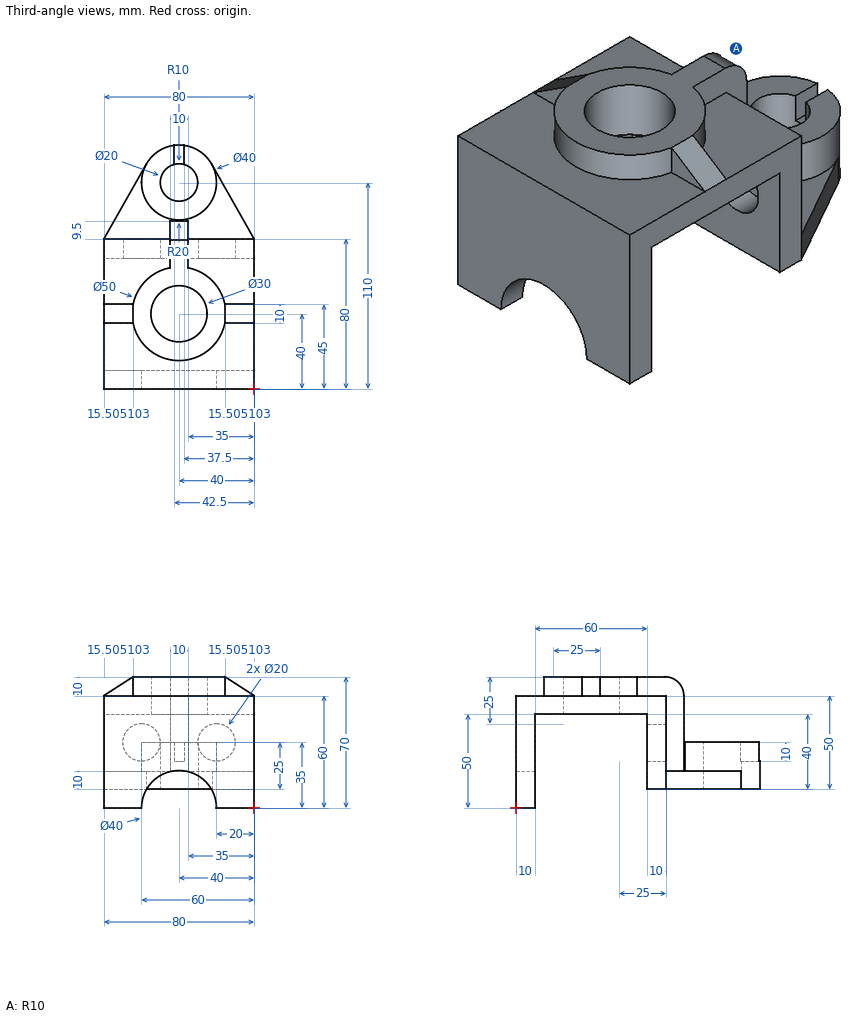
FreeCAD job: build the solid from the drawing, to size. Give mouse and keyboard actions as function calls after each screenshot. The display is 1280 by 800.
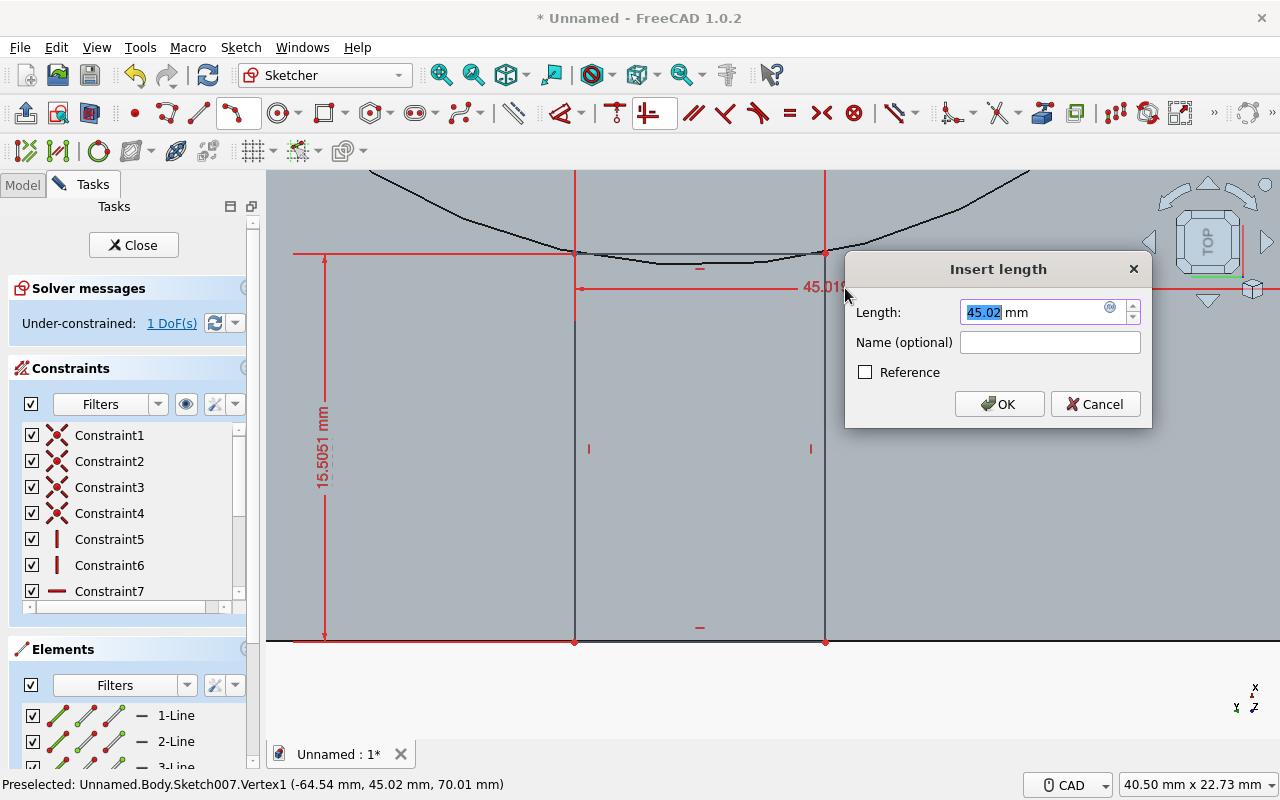
text(45)
key(Return)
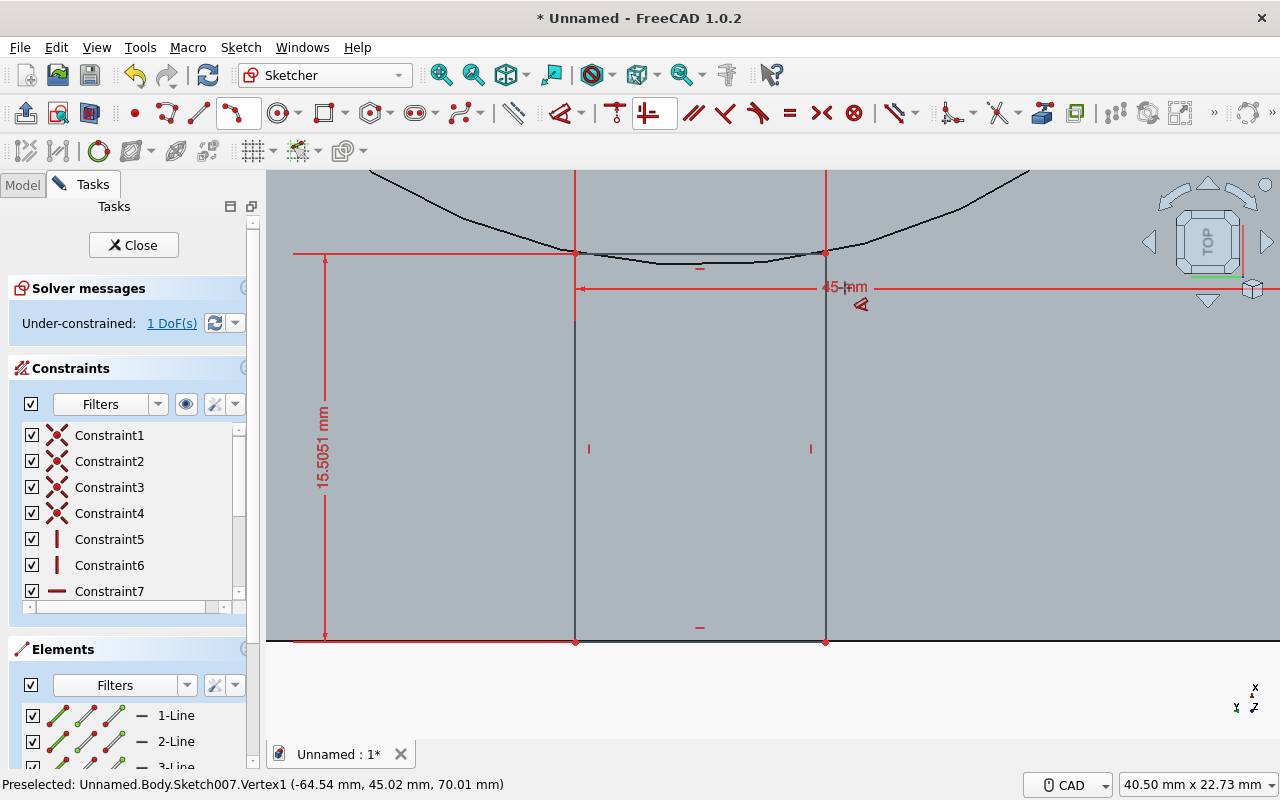
click(575, 642)
click(541, 420)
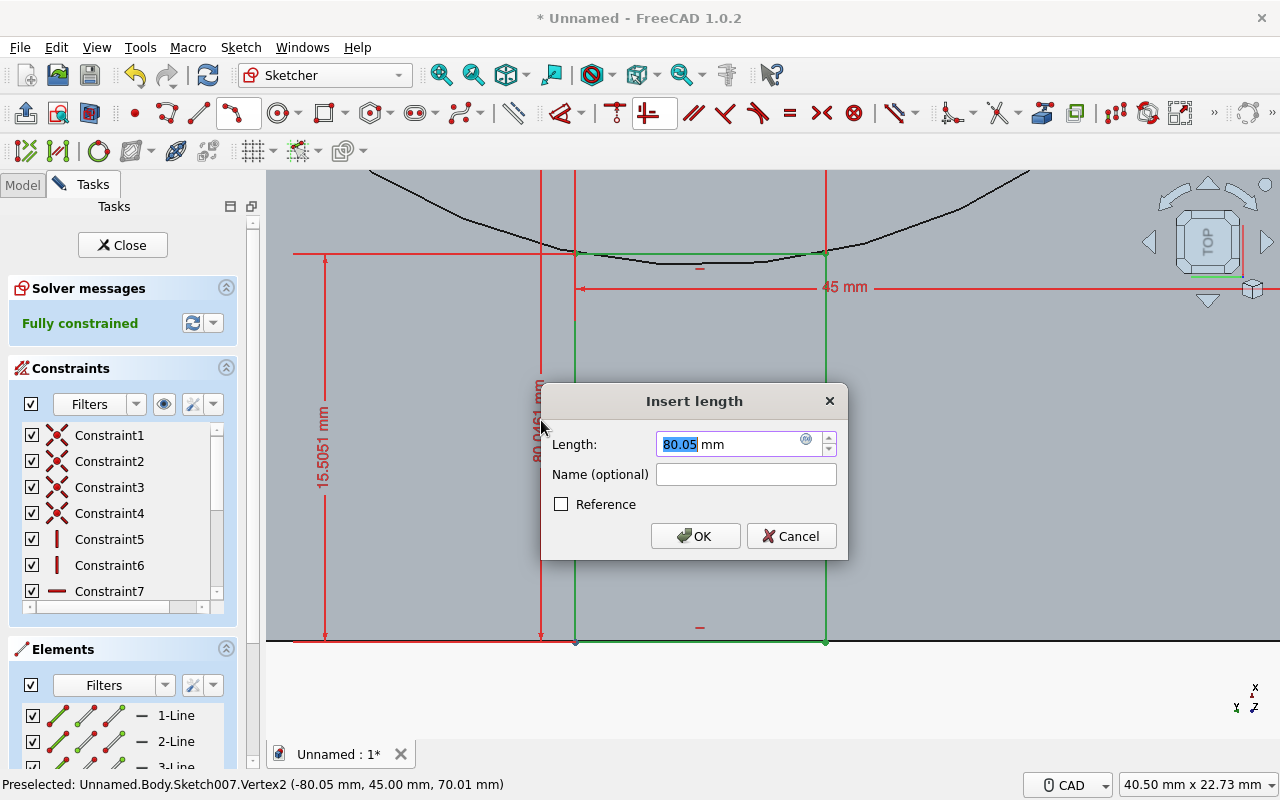
text(80)
key(Return)
key(Escape)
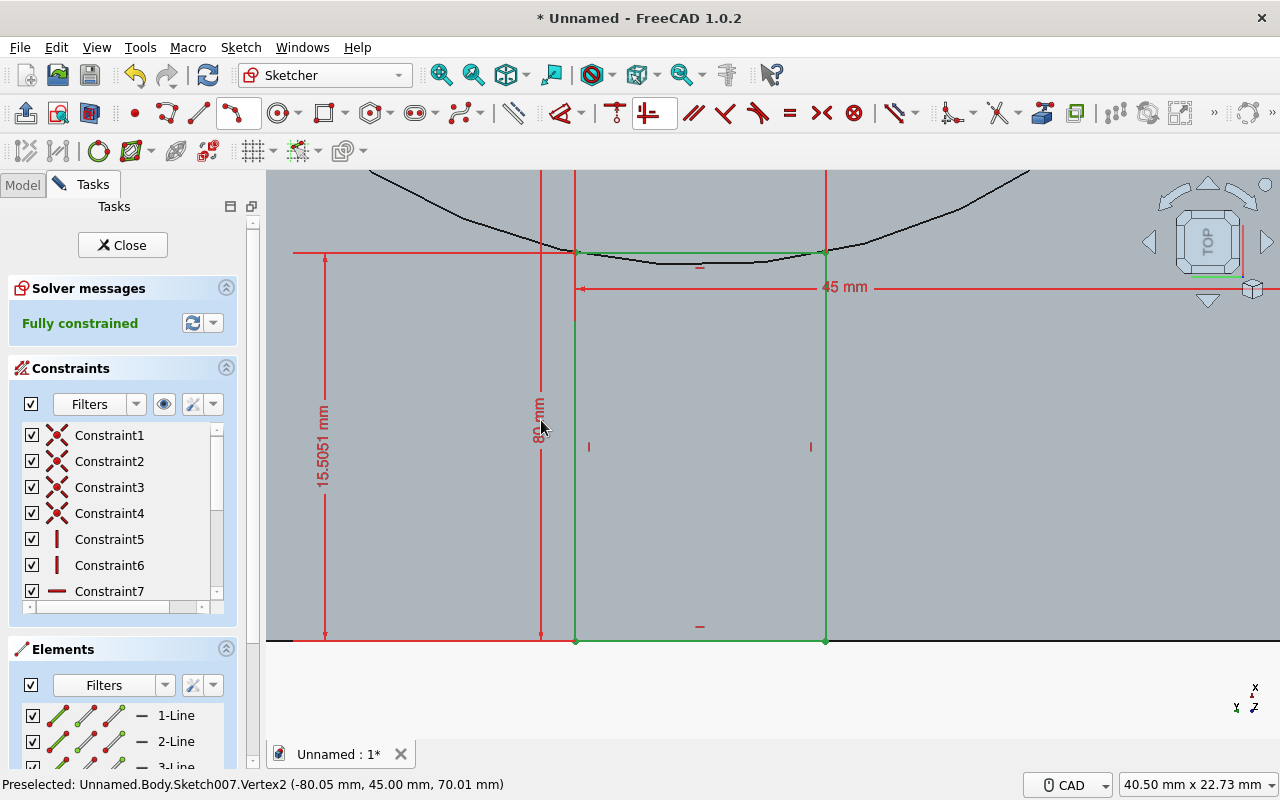
click(123, 245)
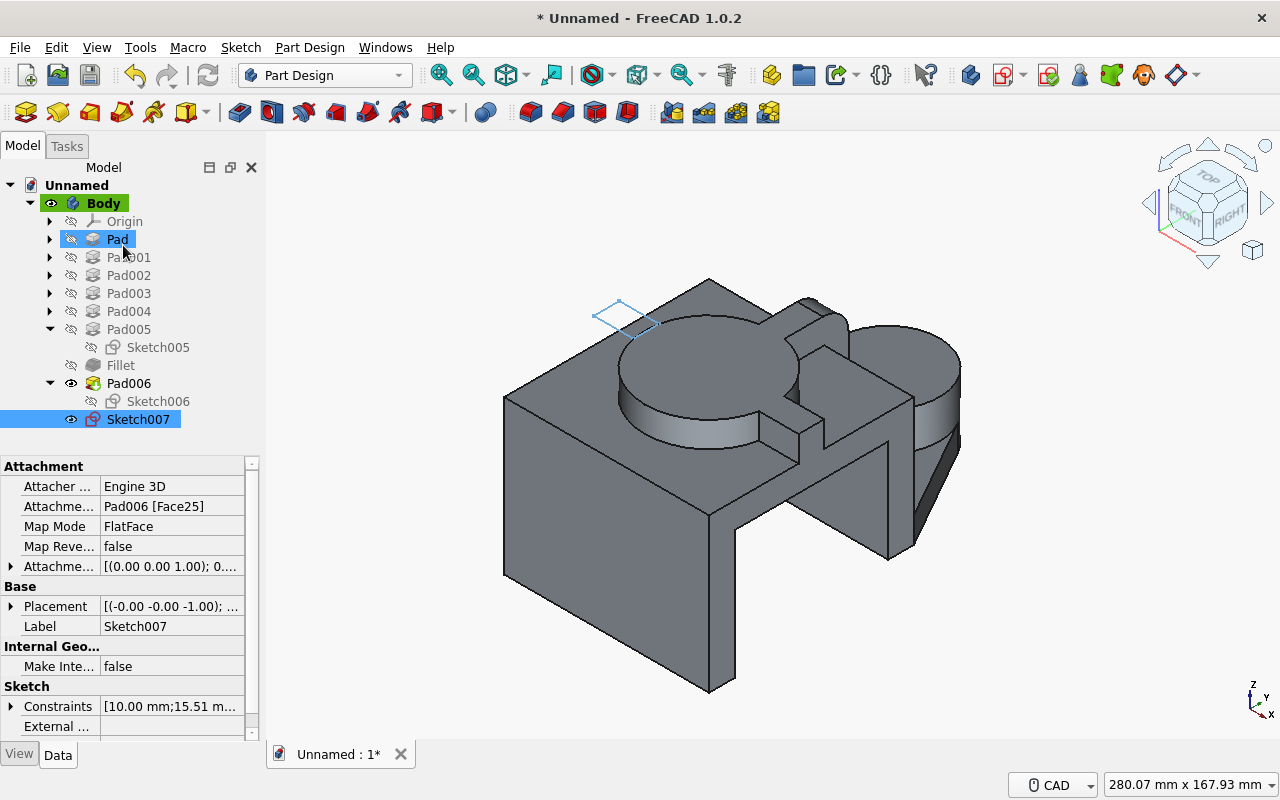
click(26, 112)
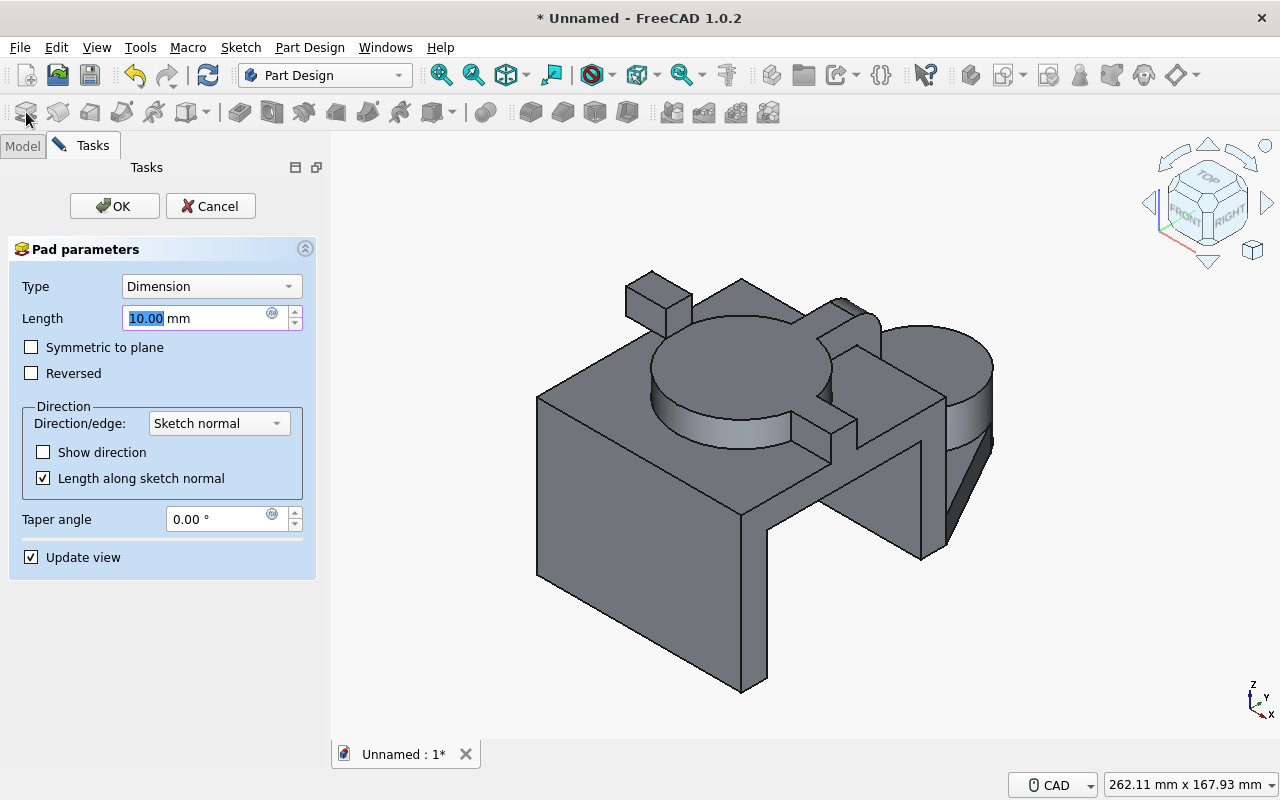
click(212, 286)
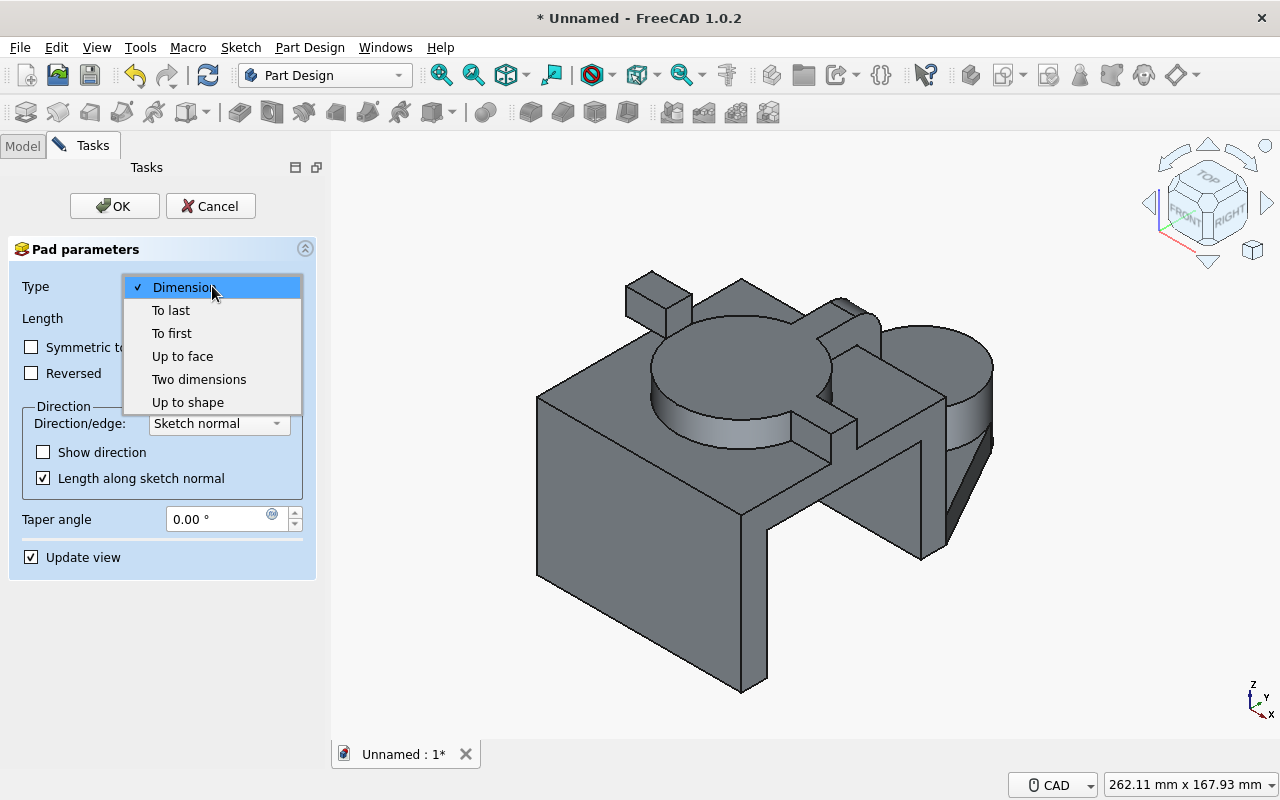
click(212, 334)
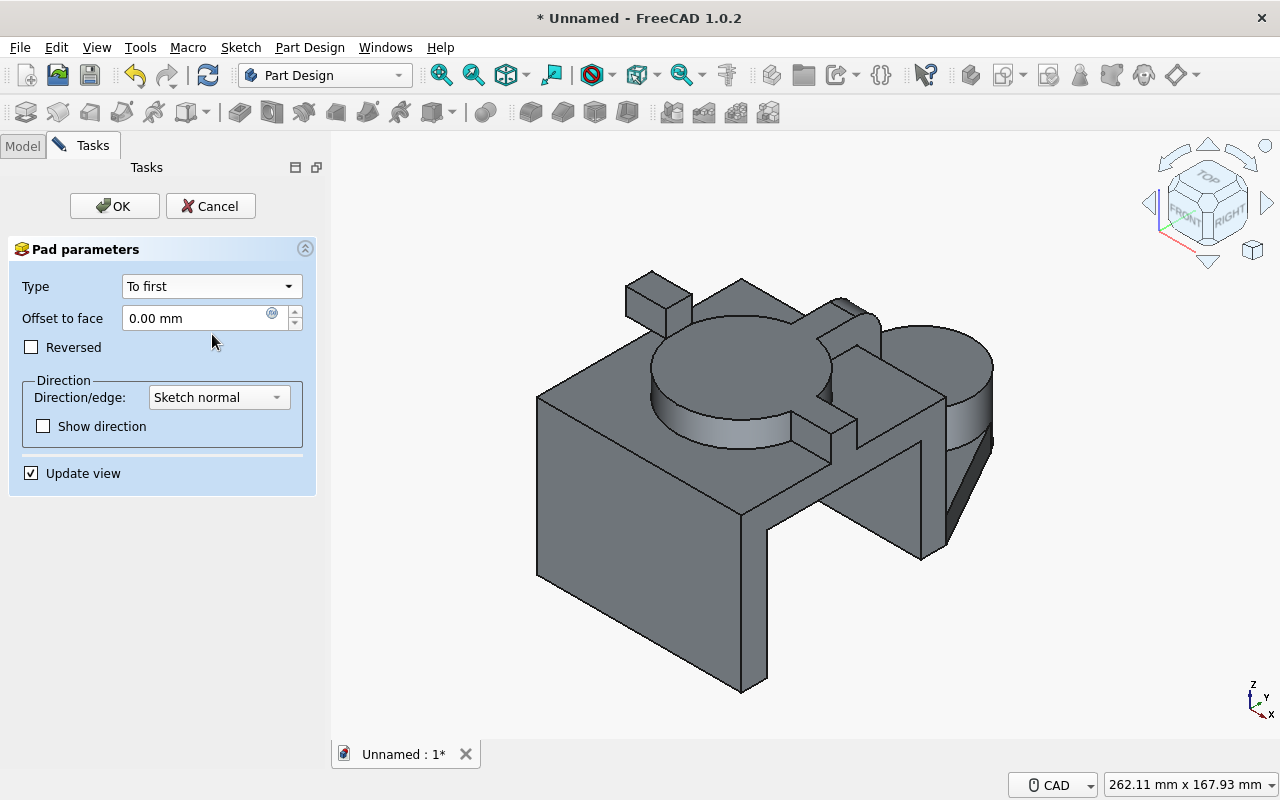
click(30, 347)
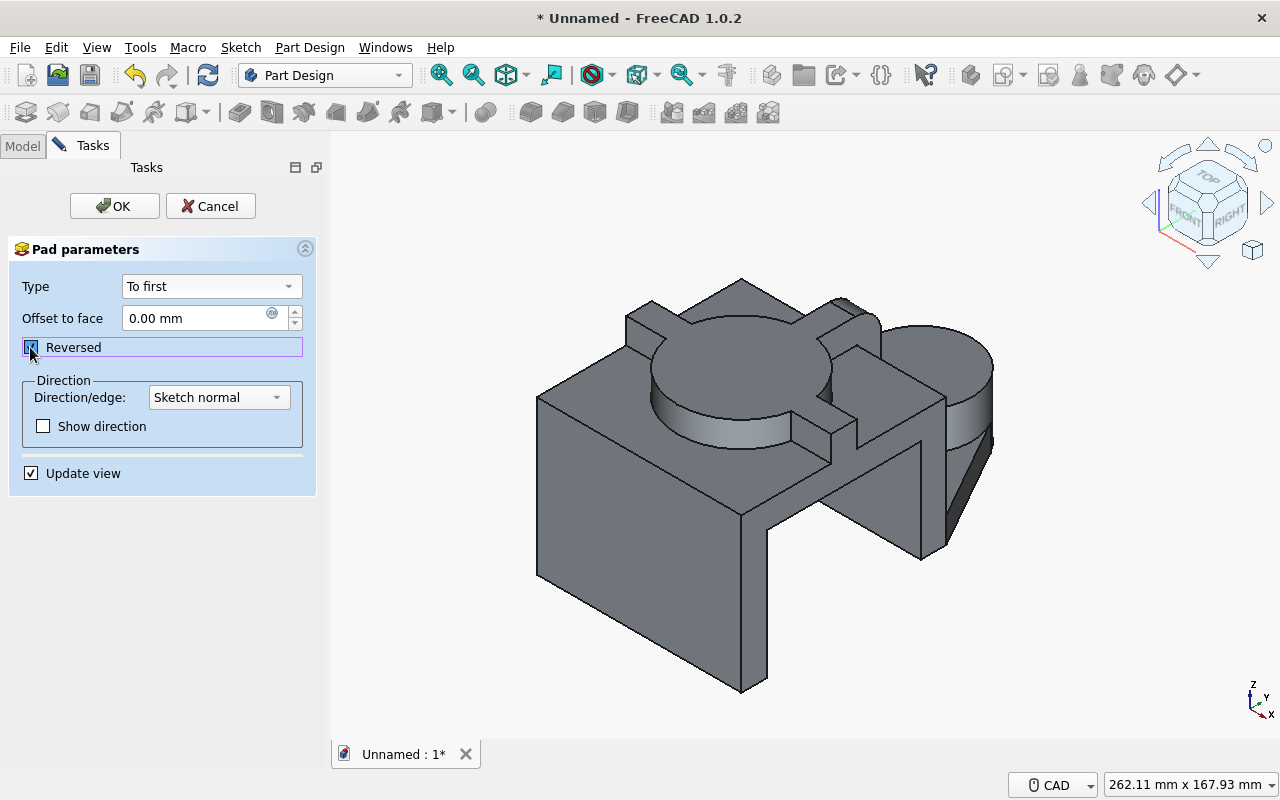
click(115, 206)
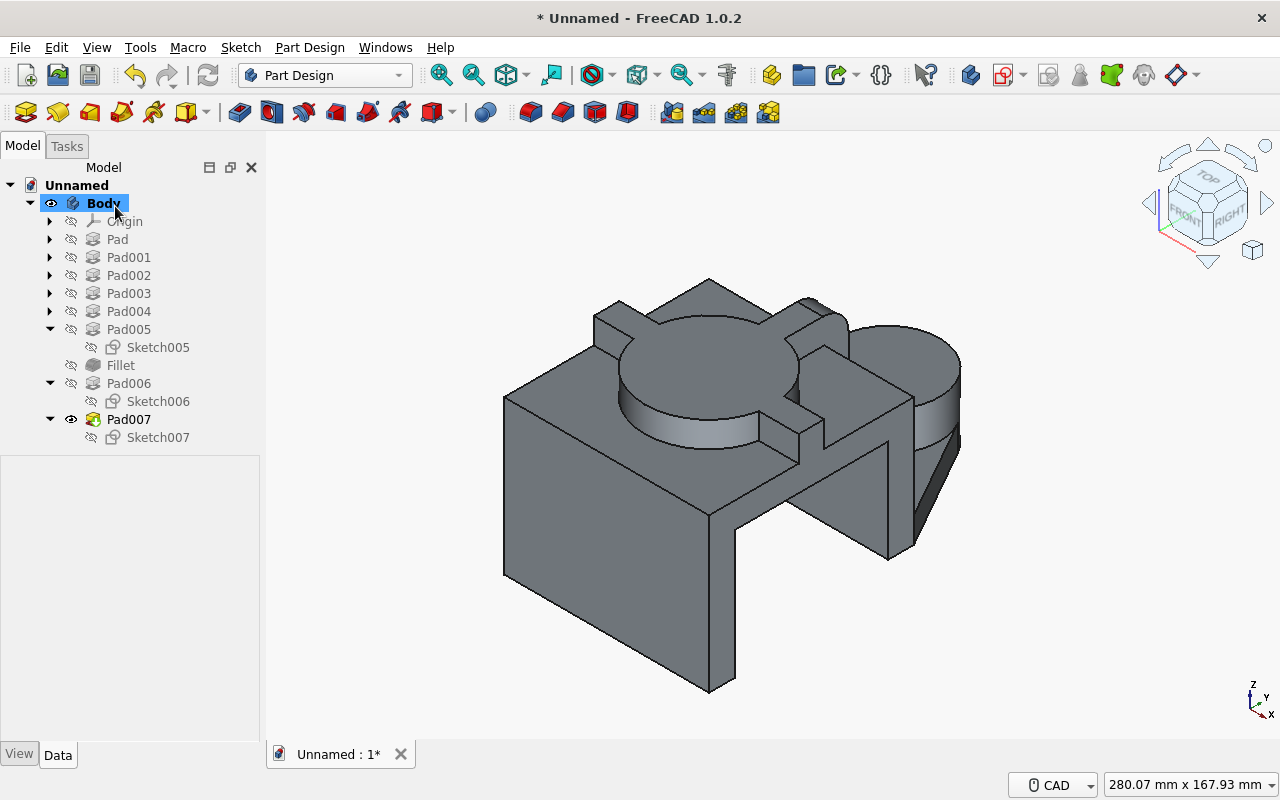
key(4)